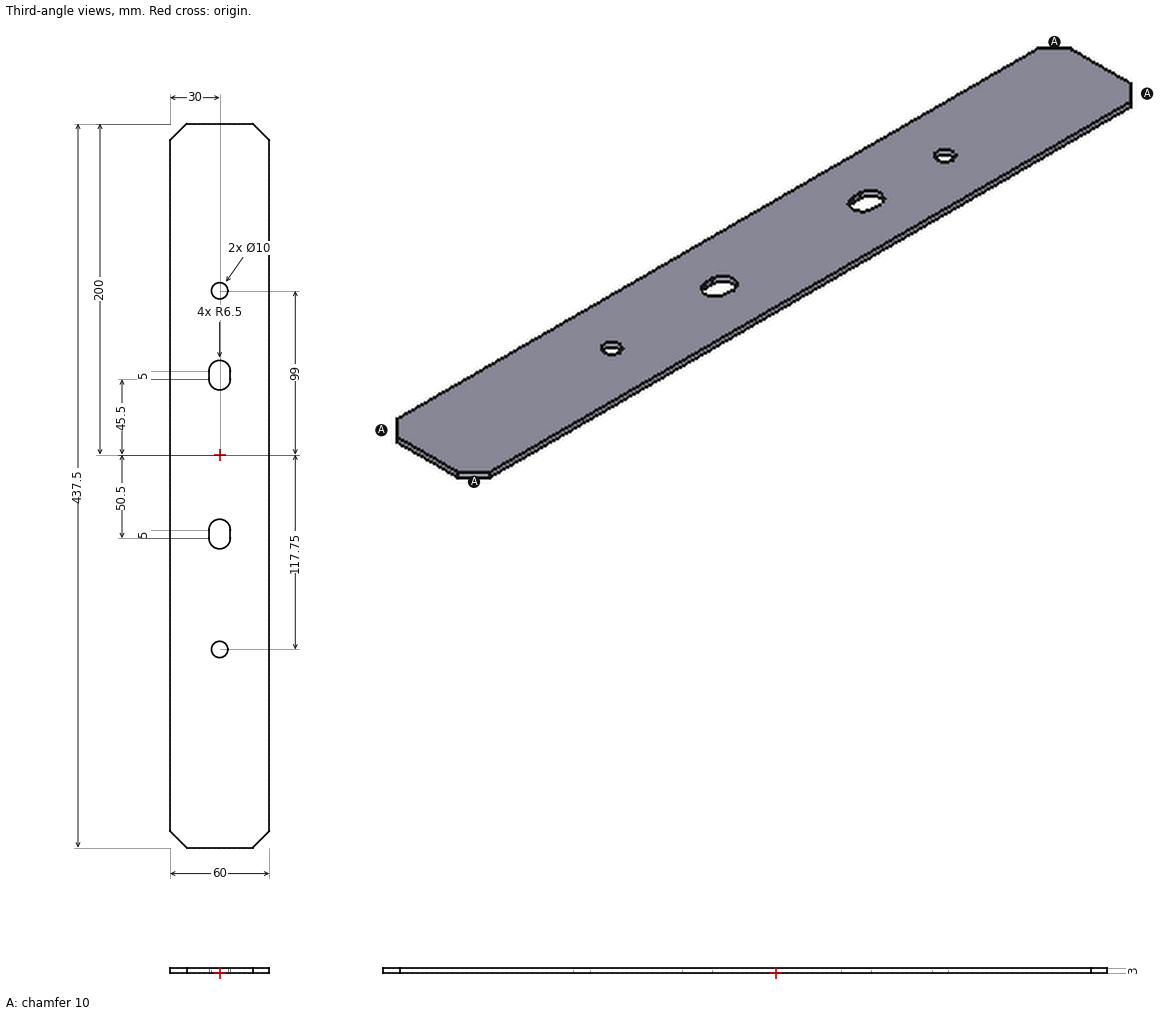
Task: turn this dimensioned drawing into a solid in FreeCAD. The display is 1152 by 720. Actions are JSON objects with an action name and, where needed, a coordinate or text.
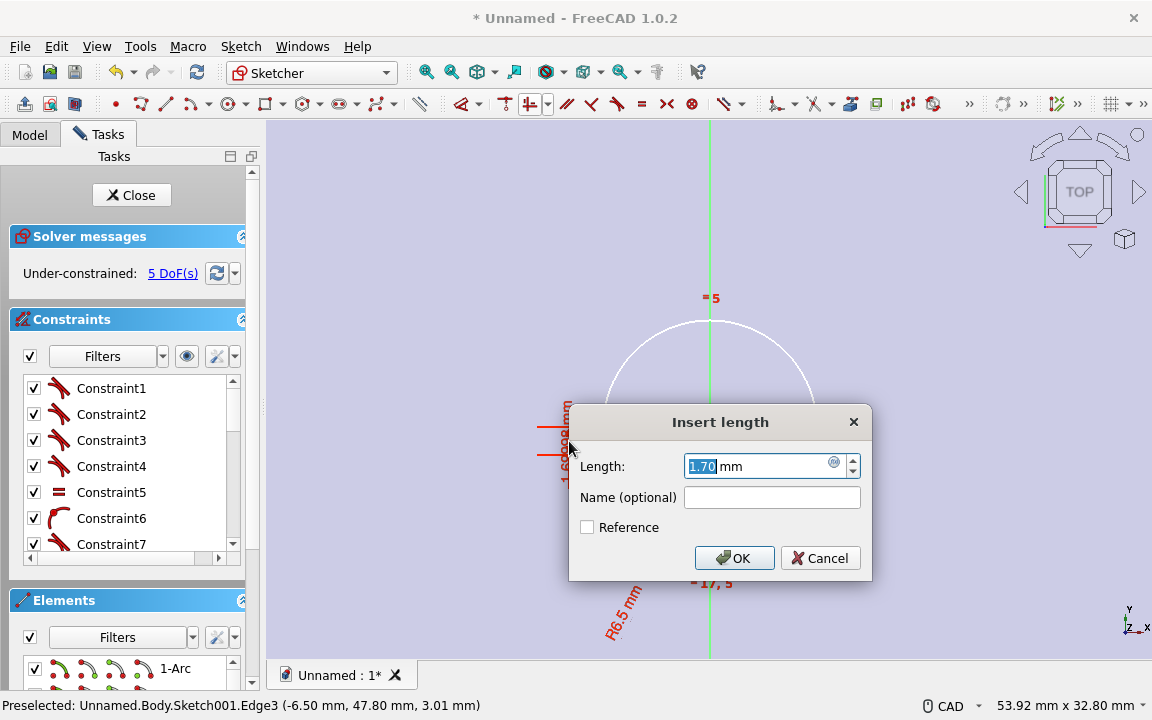
{"action": "type", "text": "5"}
{"action": "key", "text": "Return"}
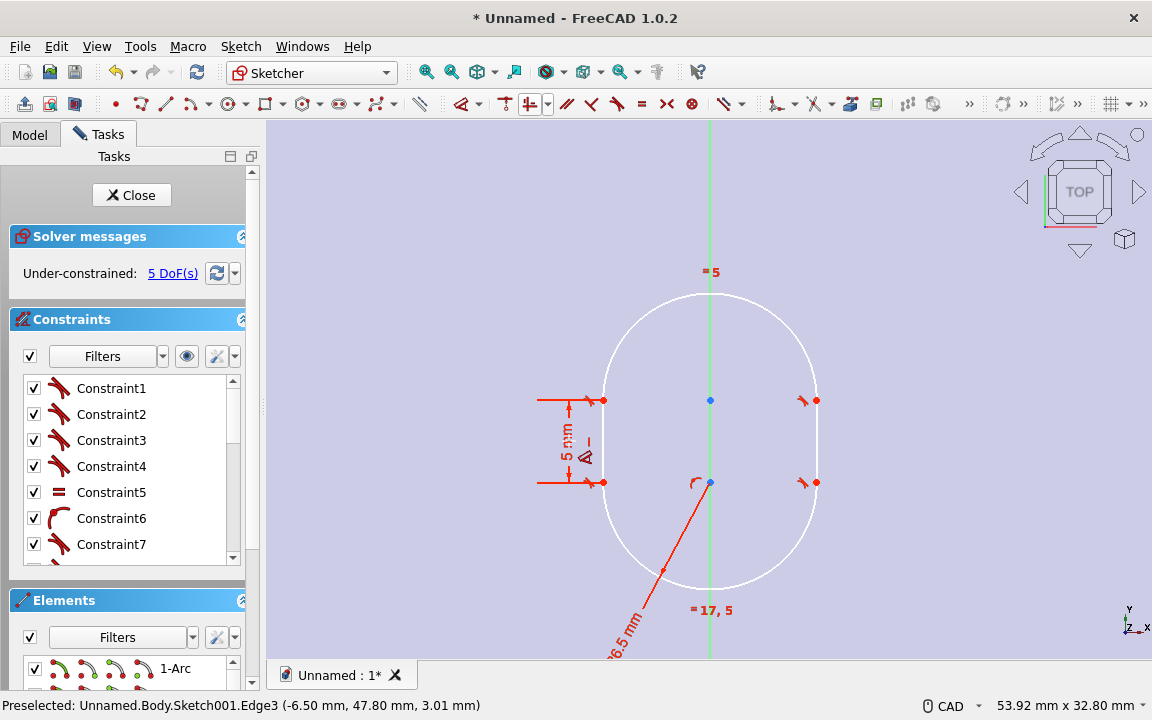
{"action": "scroll", "coordinate": [634, 291], "scroll_direction": "down", "scroll_amount": 12}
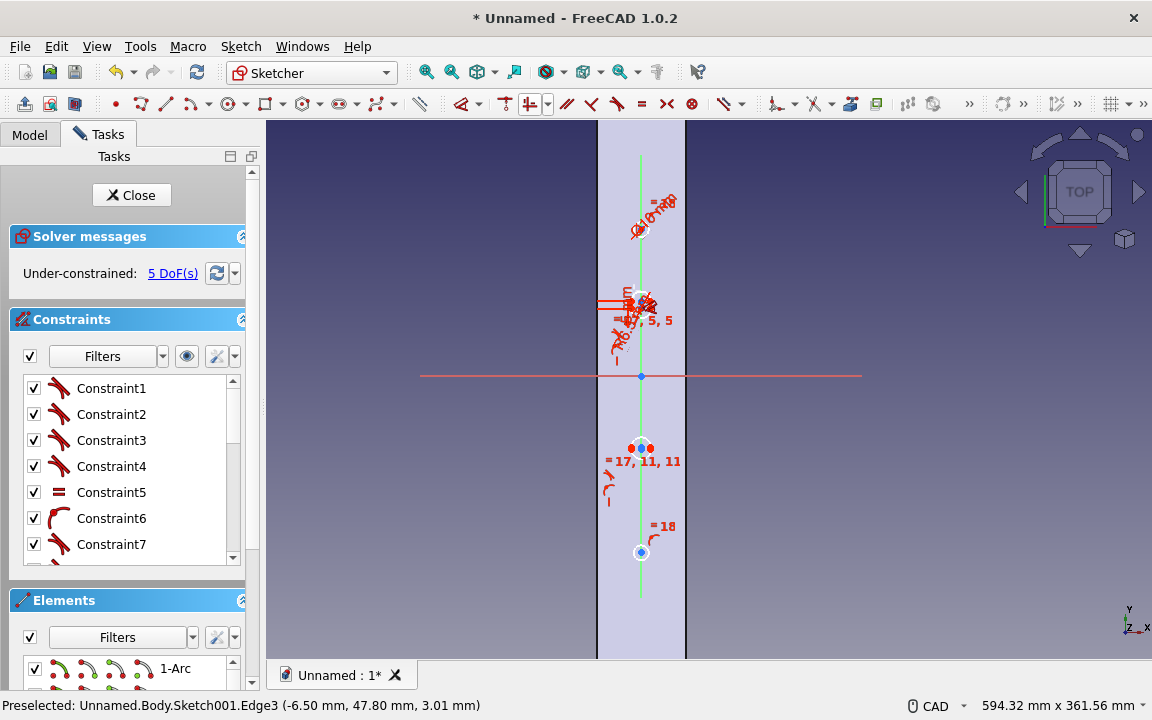
{"action": "scroll", "coordinate": [632, 448], "scroll_direction": "up", "scroll_amount": 13}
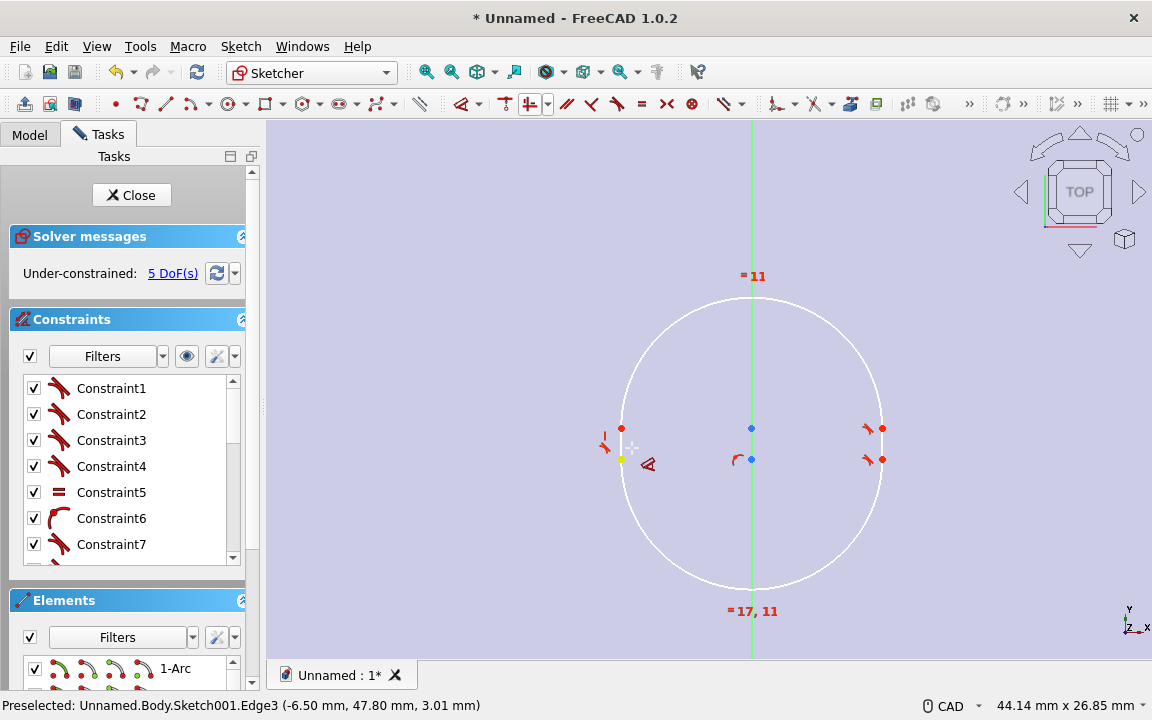
{"action": "left_click", "coordinate": [621, 447]}
{"action": "left_click", "coordinate": [587, 444]}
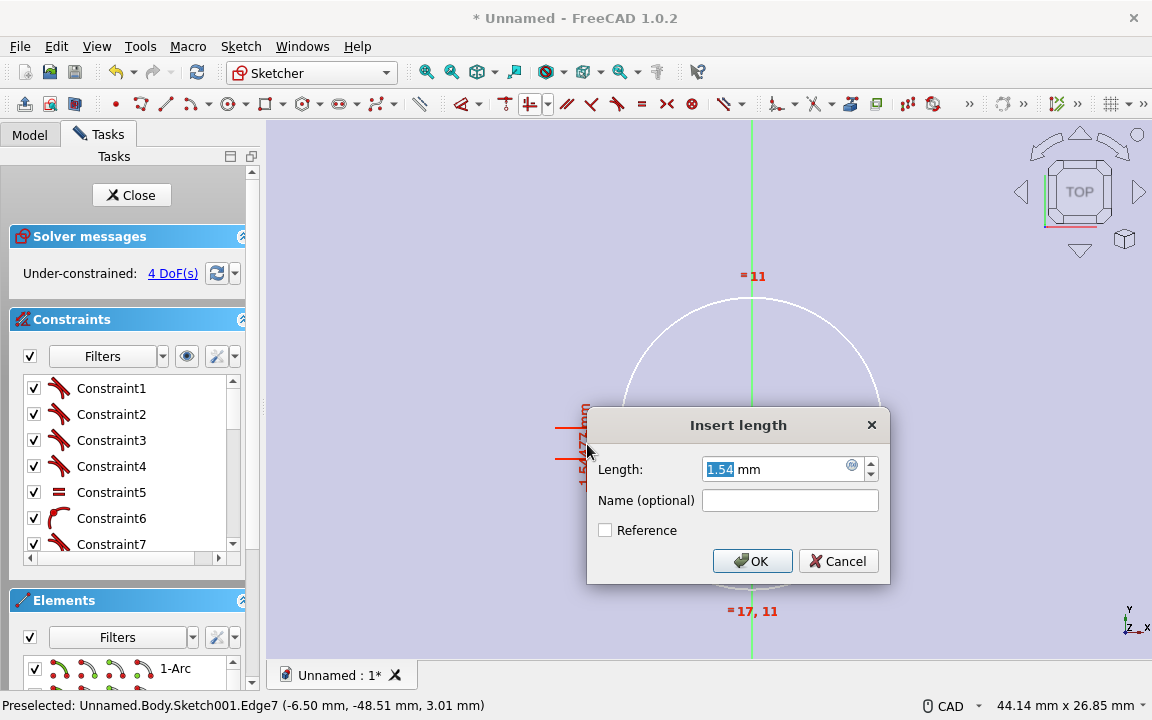
{"action": "type", "text": "5"}
{"action": "key", "text": "Return"}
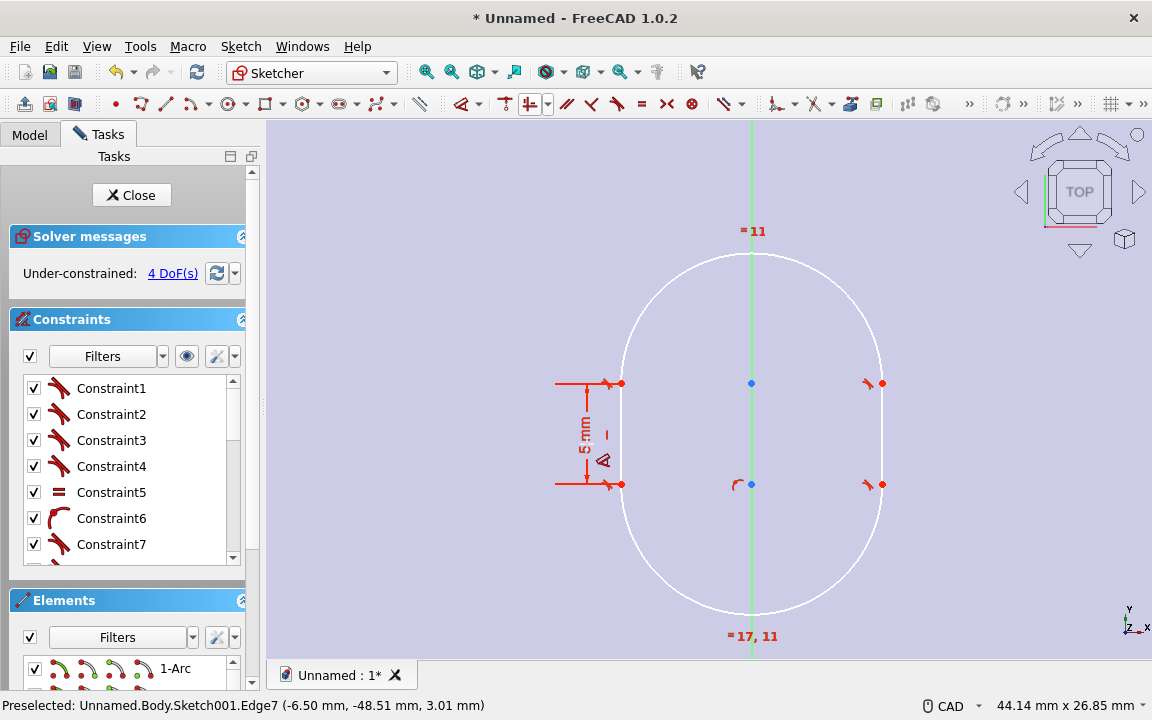
{"action": "scroll", "coordinate": [632, 448], "scroll_direction": "down", "scroll_amount": 13}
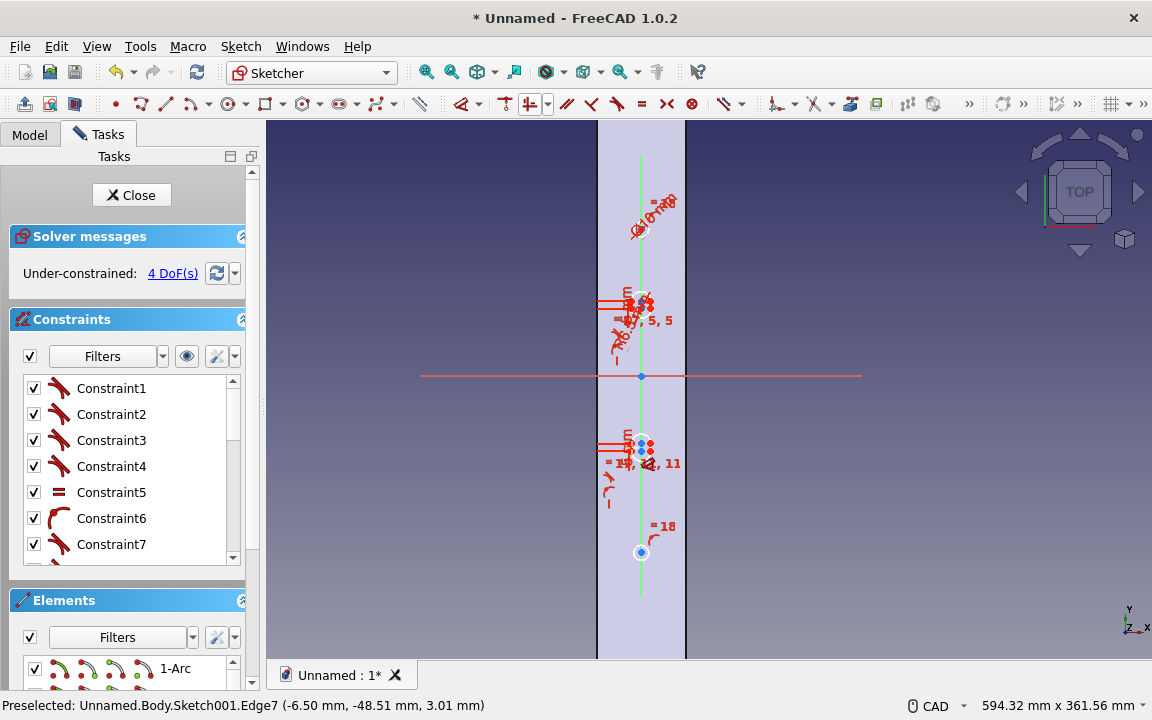
{"action": "left_click", "coordinate": [641, 230]}
{"action": "left_click", "coordinate": [675, 269]}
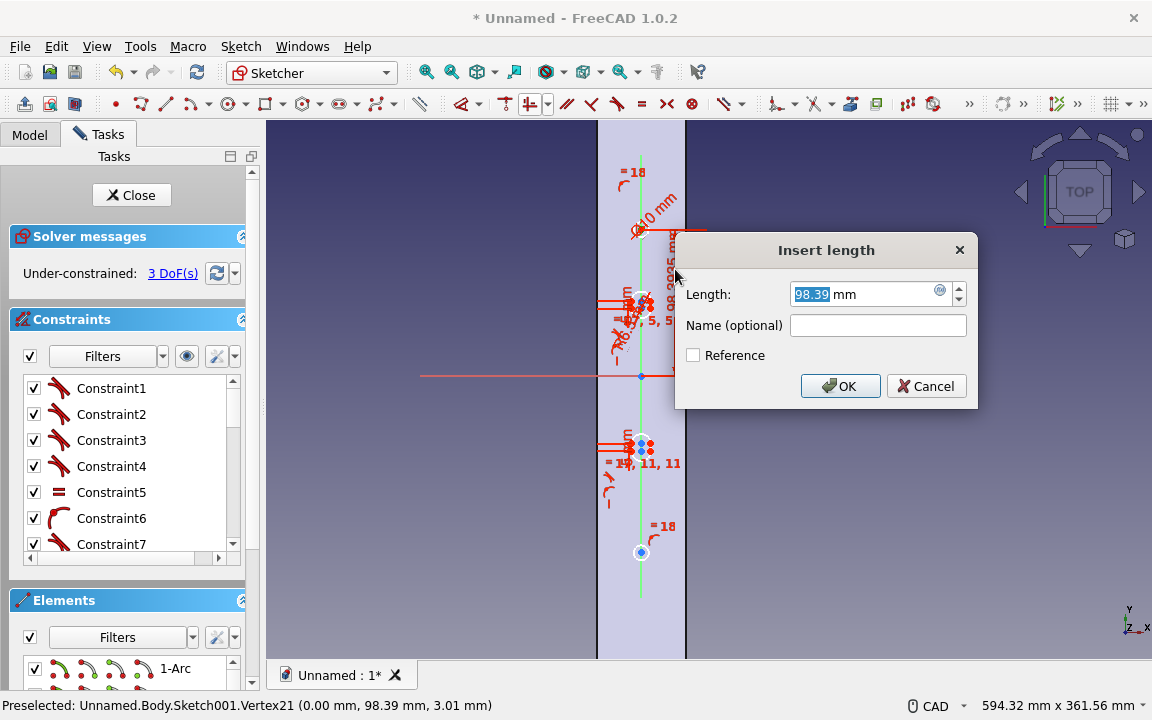
{"action": "type", "text": "99"}
{"action": "key", "text": "Return"}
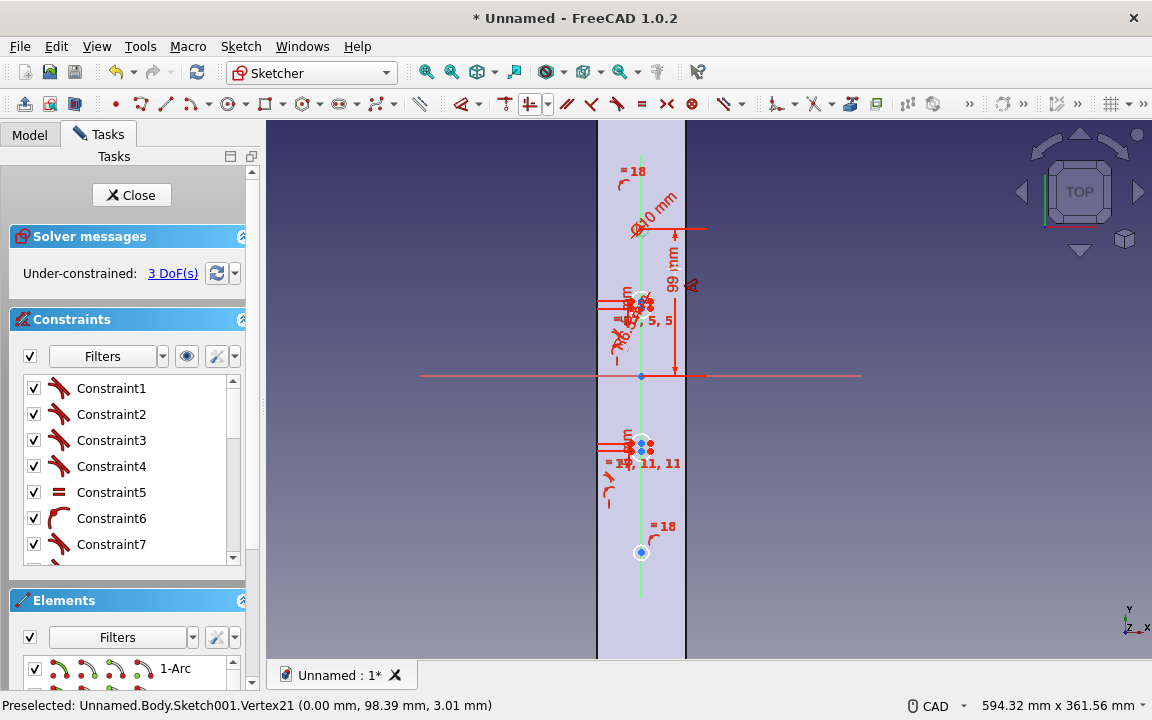
{"action": "scroll", "coordinate": [632, 309], "scroll_direction": "up", "scroll_amount": 3}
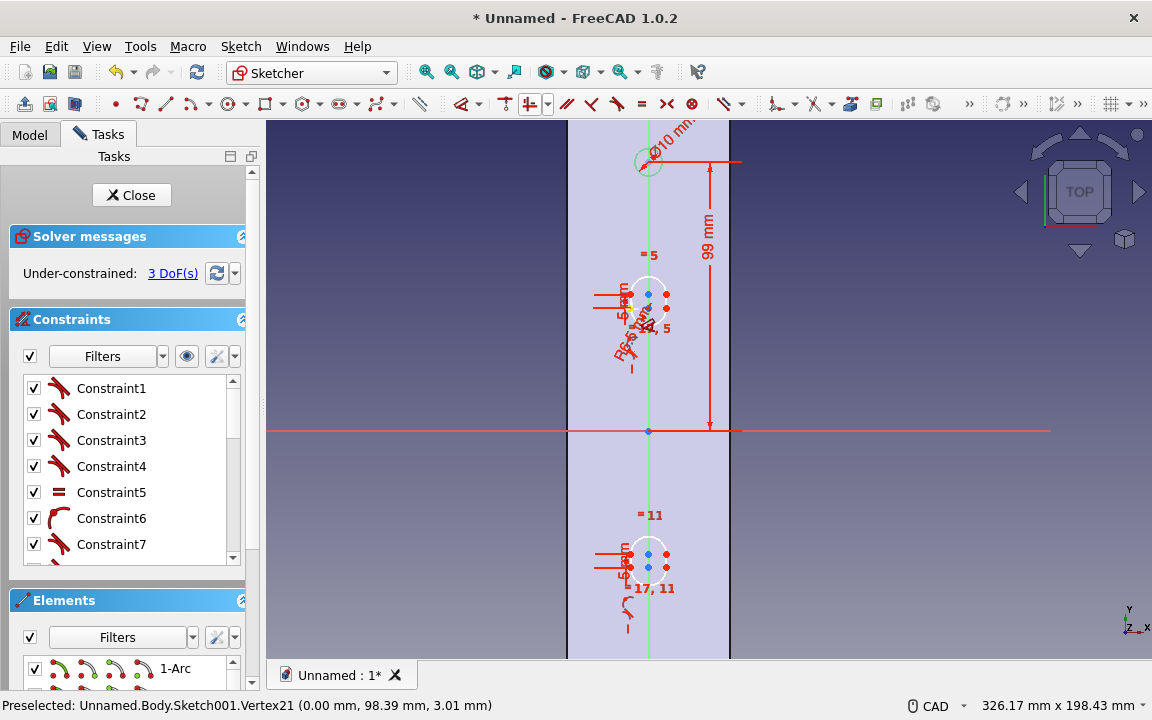
{"action": "left_click", "coordinate": [631, 308]}
{"action": "left_click", "coordinate": [597, 370]}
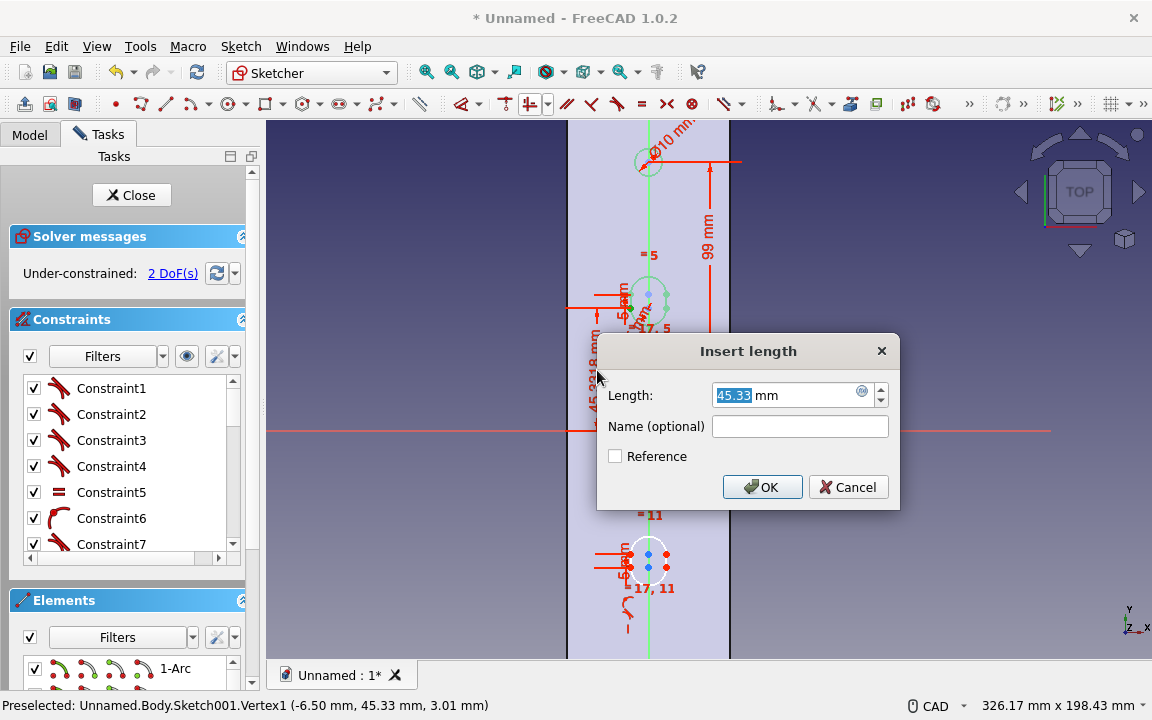
{"action": "type", "text": "45.5"}
{"action": "key", "text": "Return"}